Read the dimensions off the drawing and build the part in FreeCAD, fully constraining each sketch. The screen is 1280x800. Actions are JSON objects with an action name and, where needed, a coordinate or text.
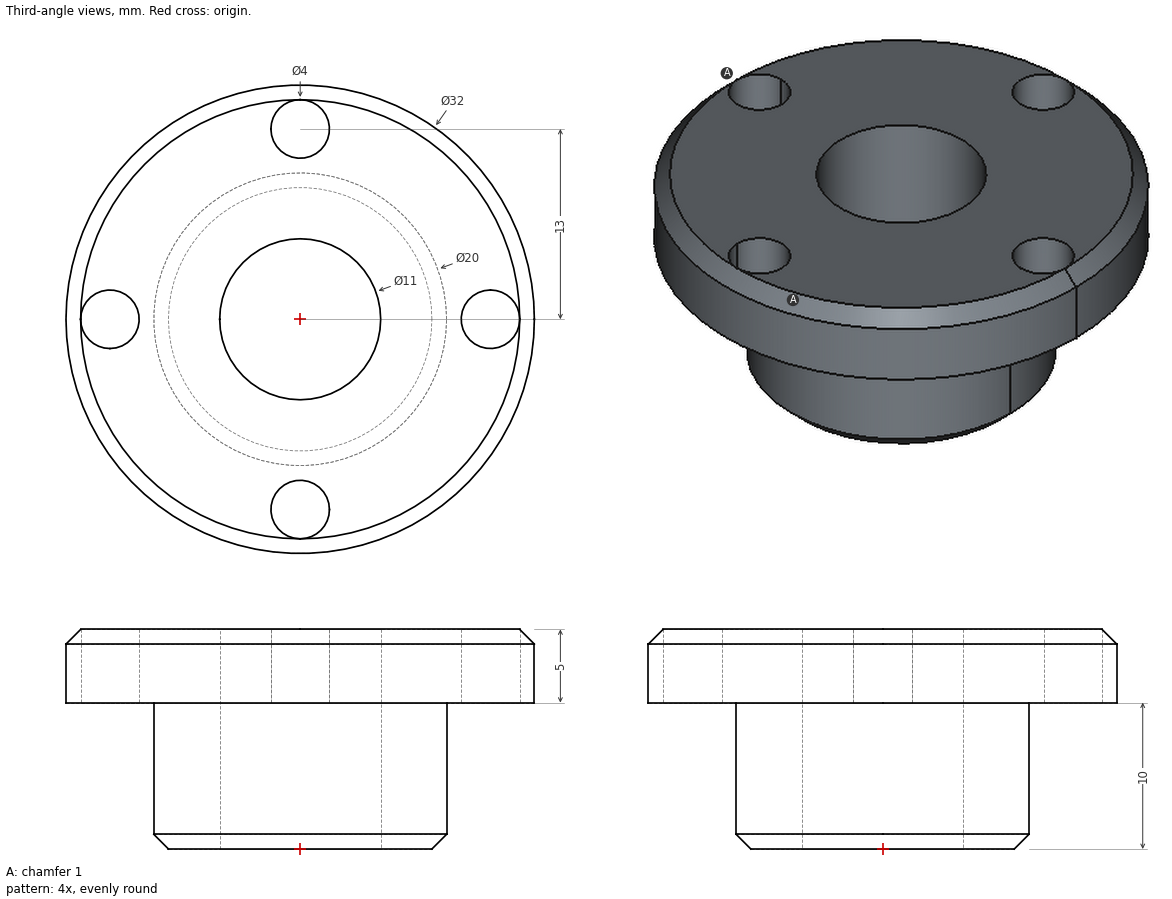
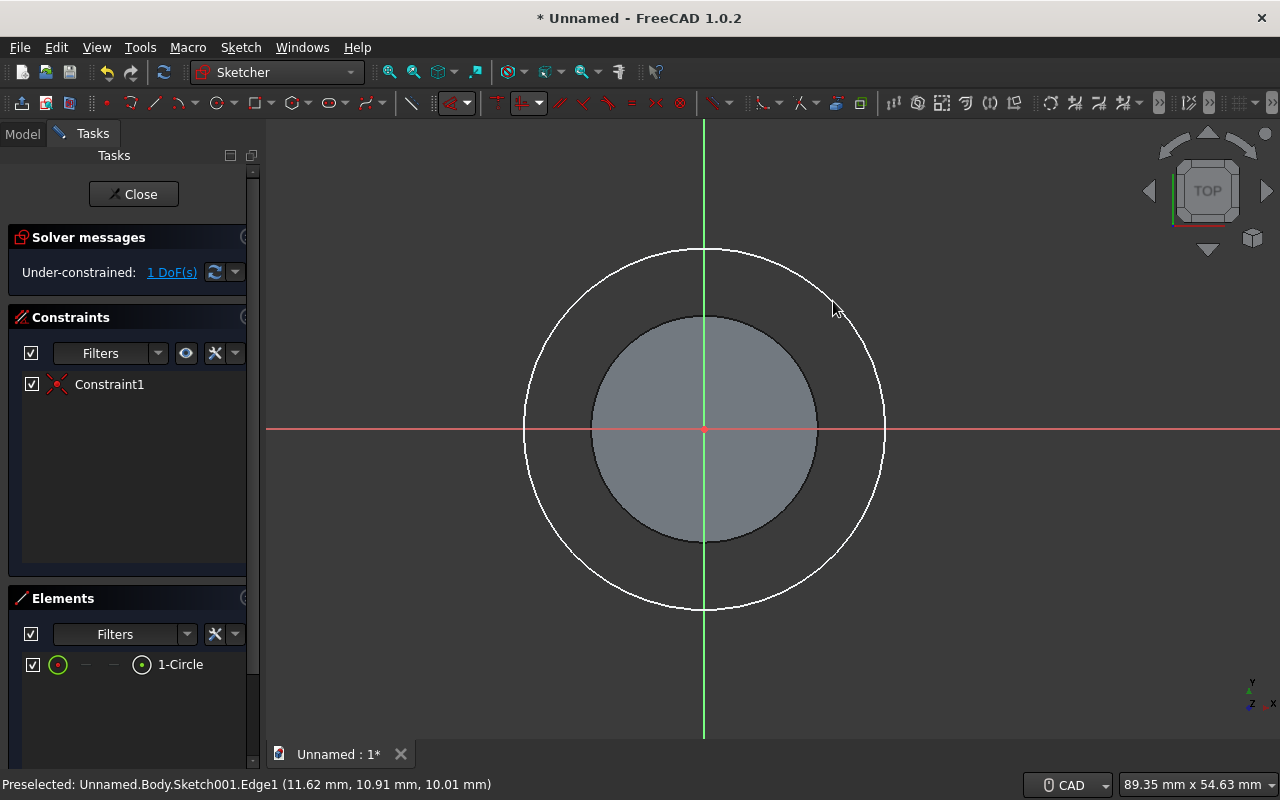
{"action": "left_click", "coordinate": [832, 301]}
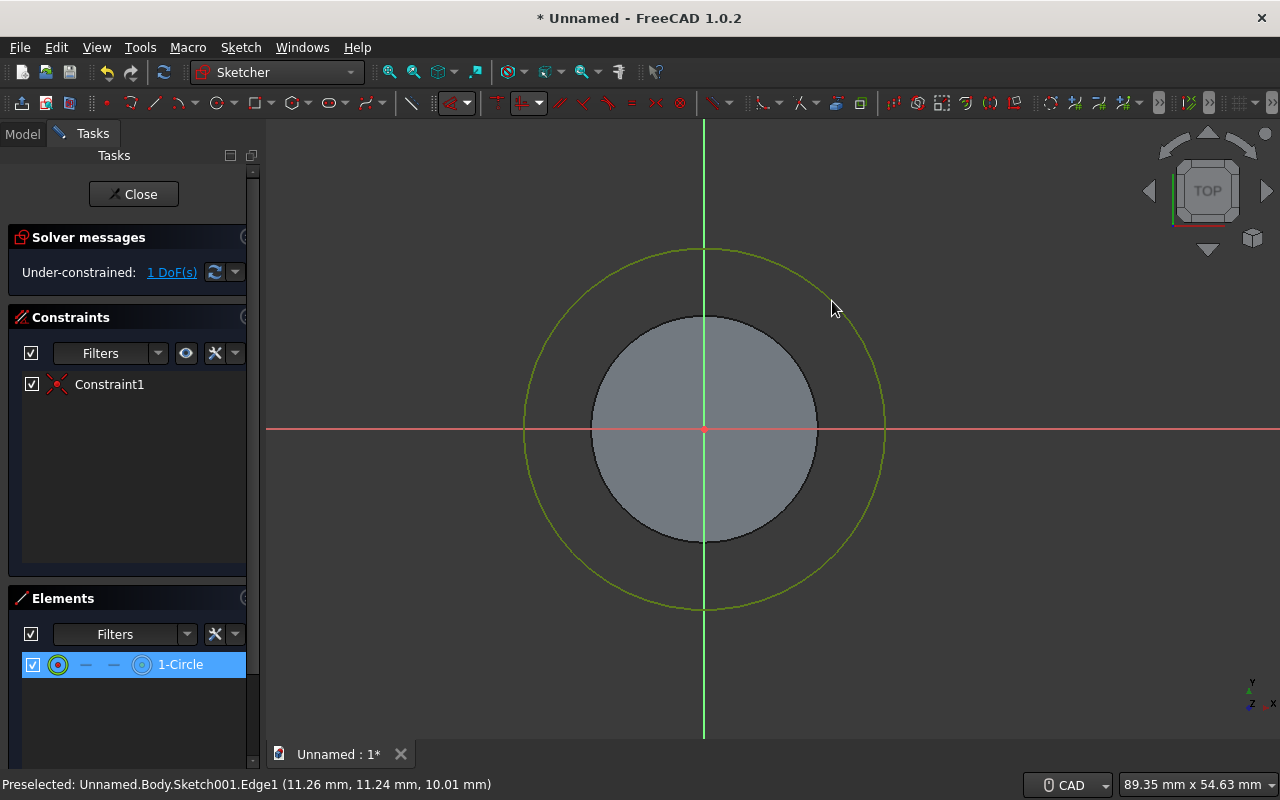
{"action": "key", "text": "k o"}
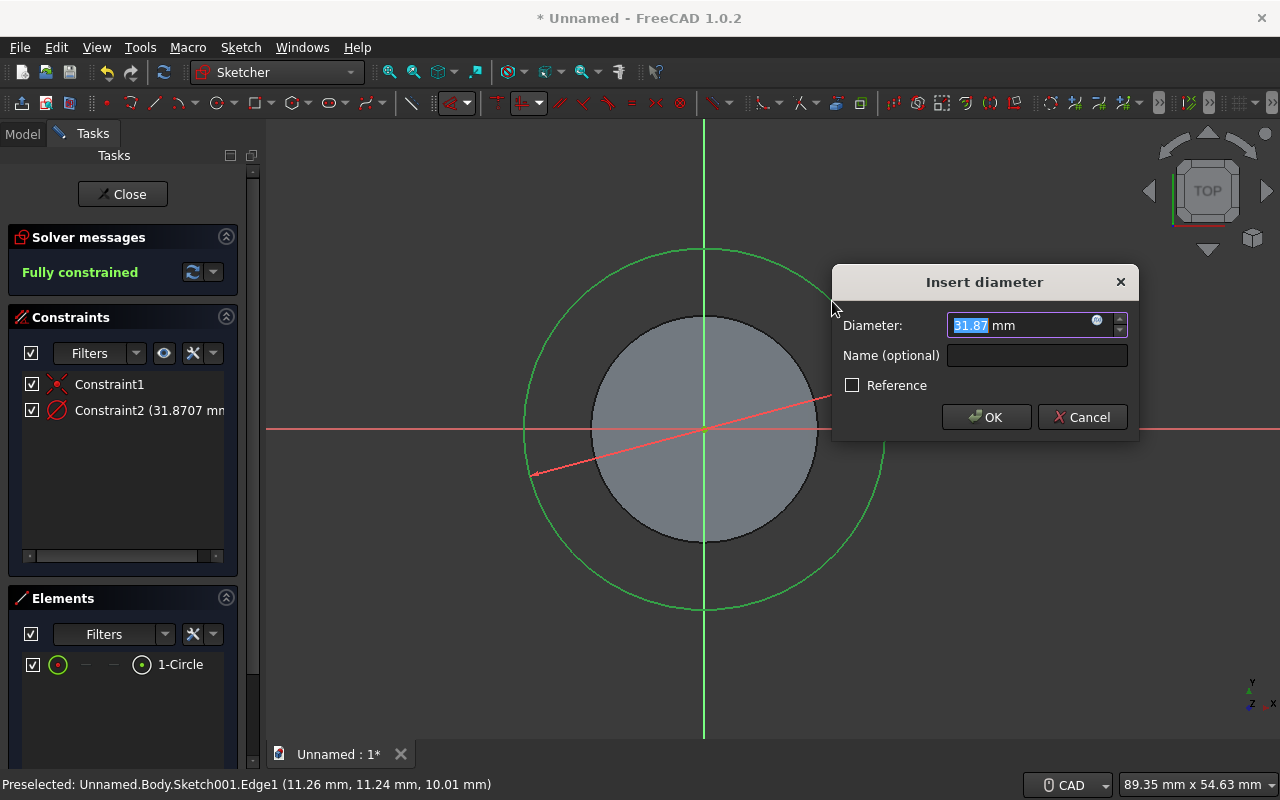
{"action": "type", "text": "32"}
{"action": "key", "text": "Return"}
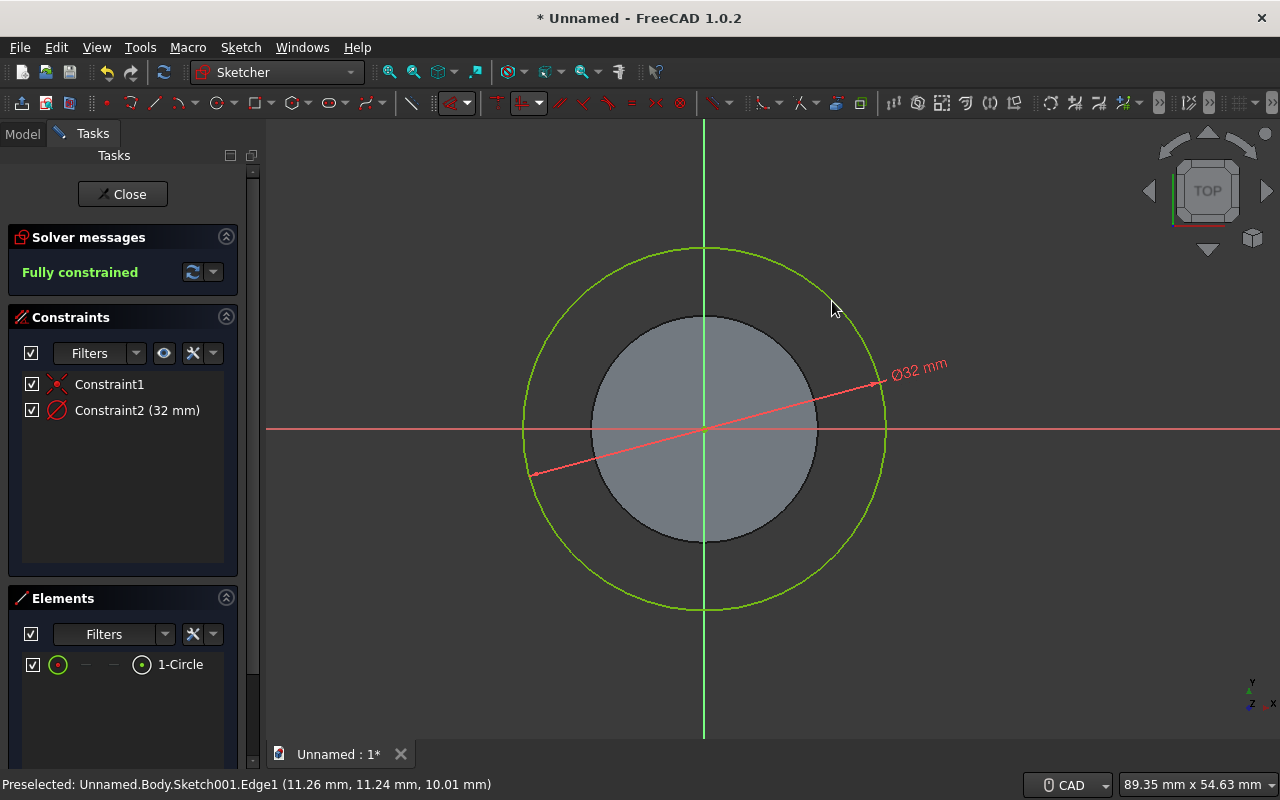
{"action": "left_click", "coordinate": [123, 194]}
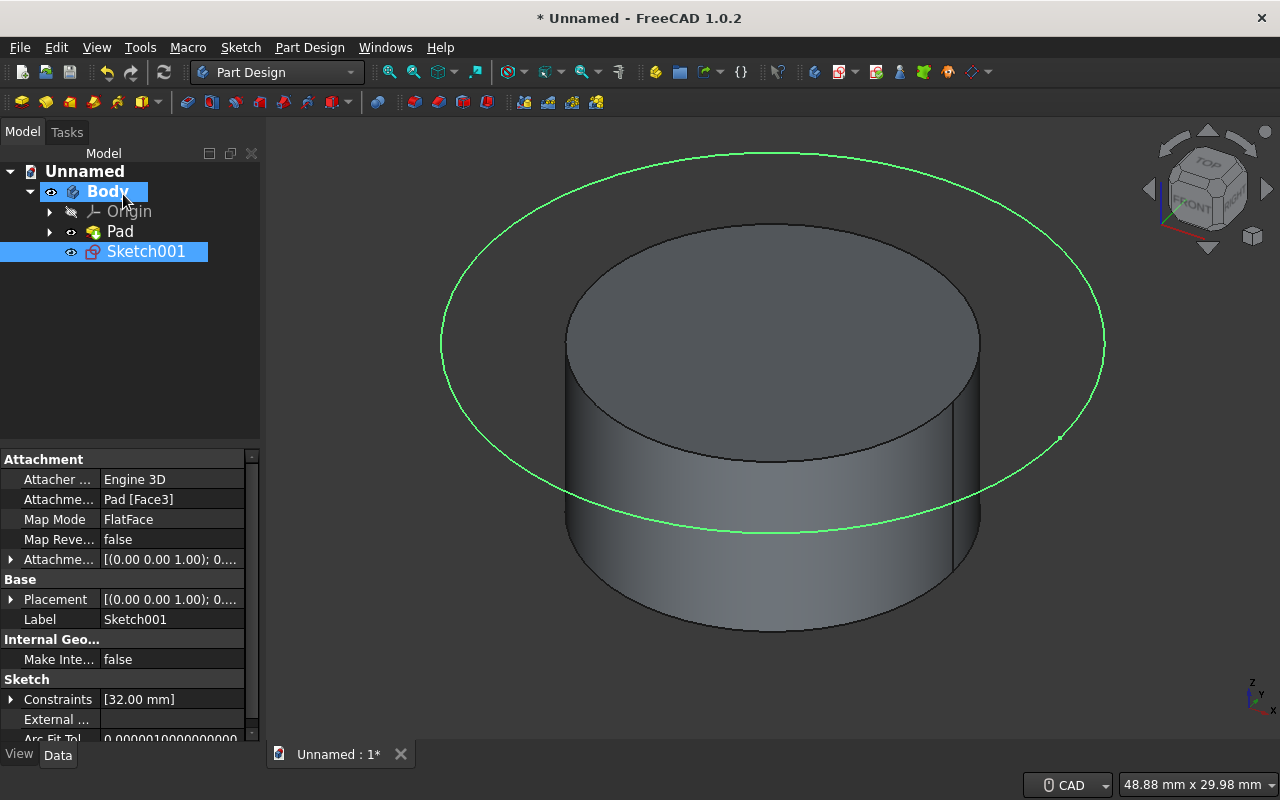
{"action": "left_click", "coordinate": [22, 102]}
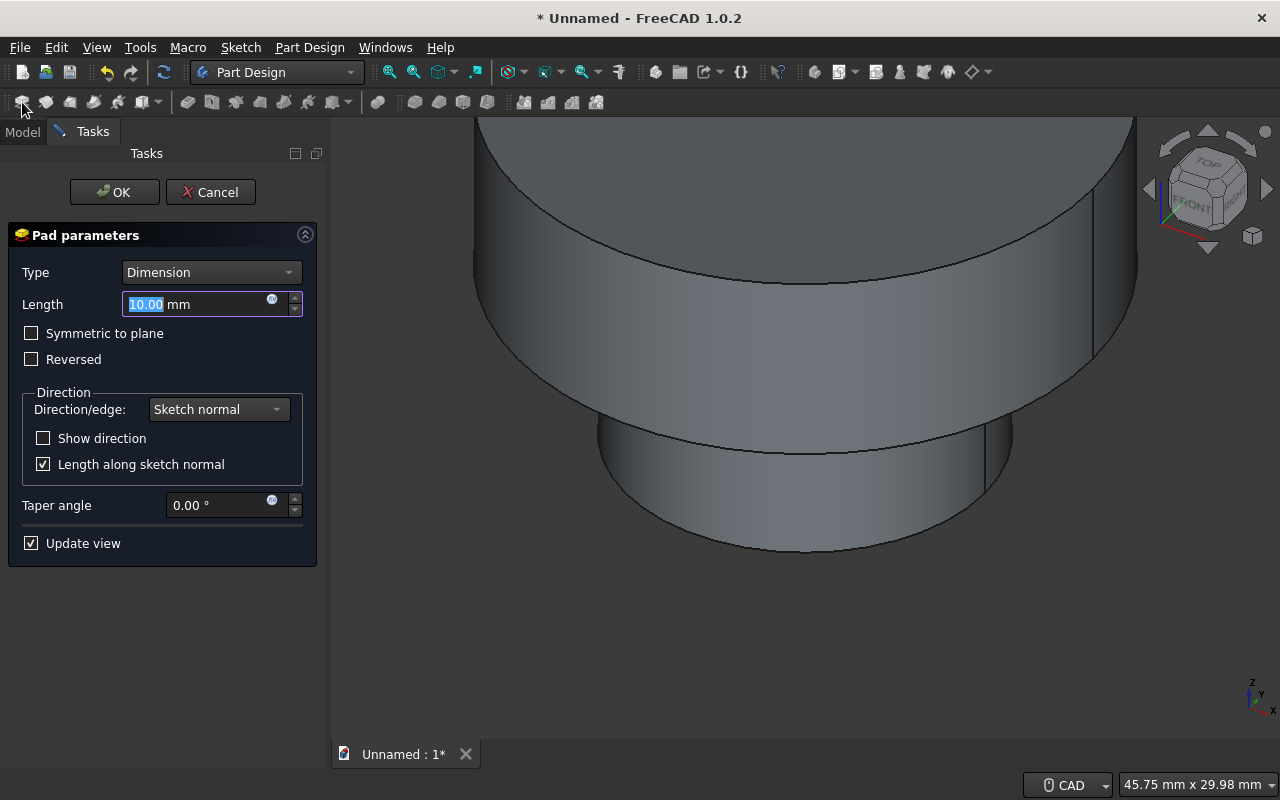
{"action": "type", "text": "5"}
{"action": "key", "text": "Tab"}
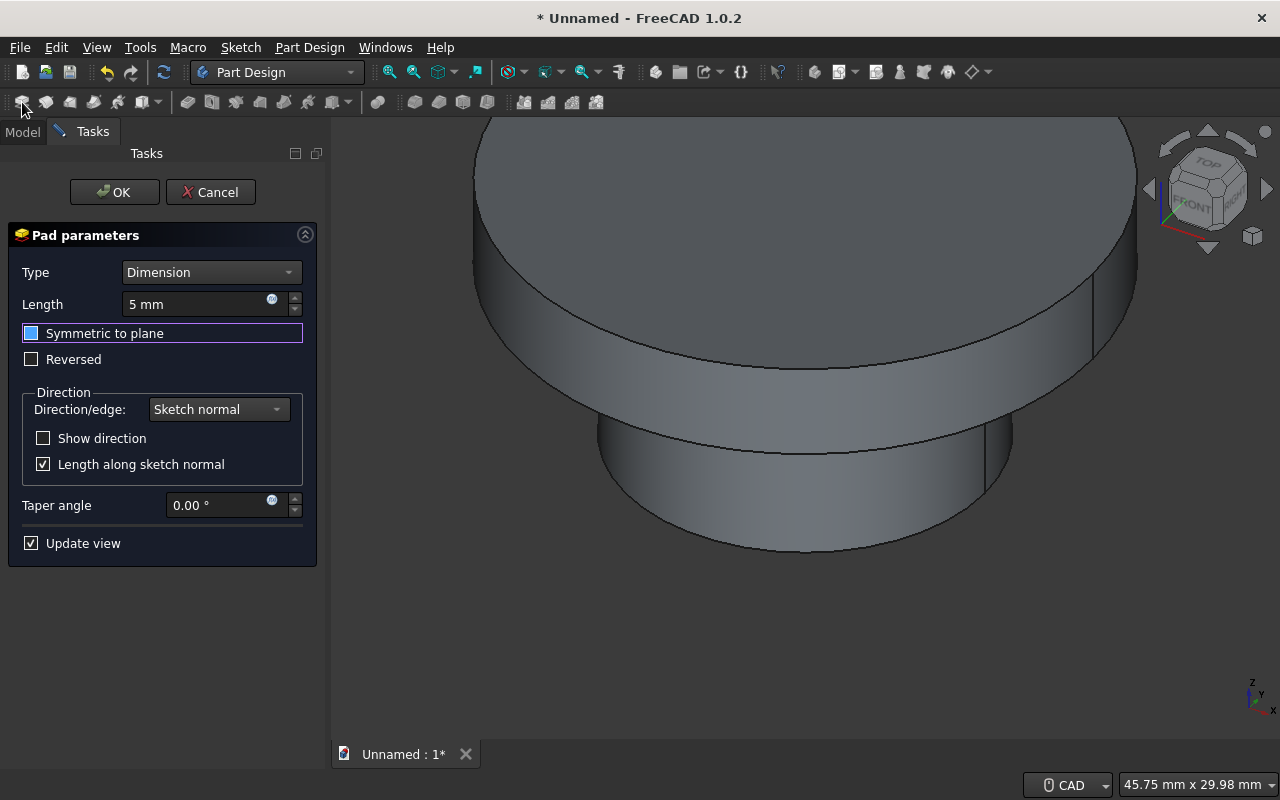
{"action": "left_click", "coordinate": [115, 192]}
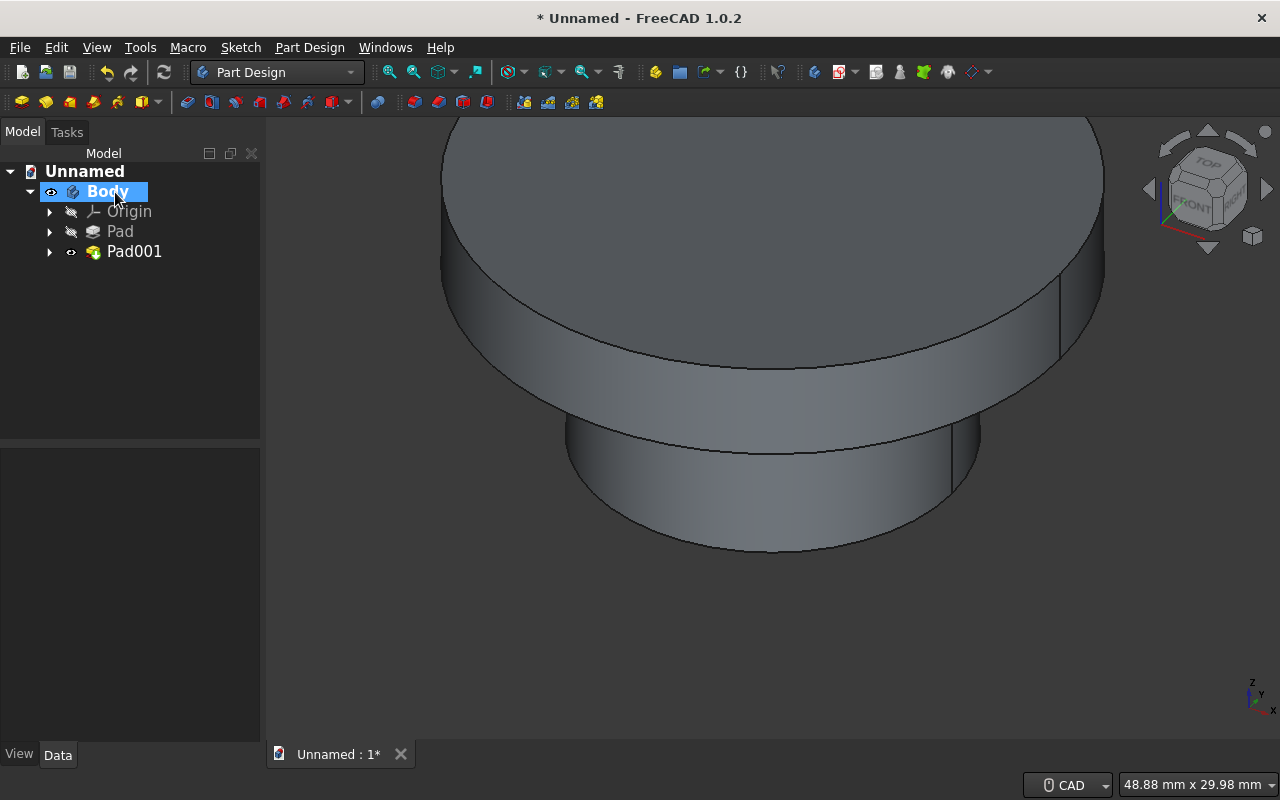
{"action": "key", "text": "v f"}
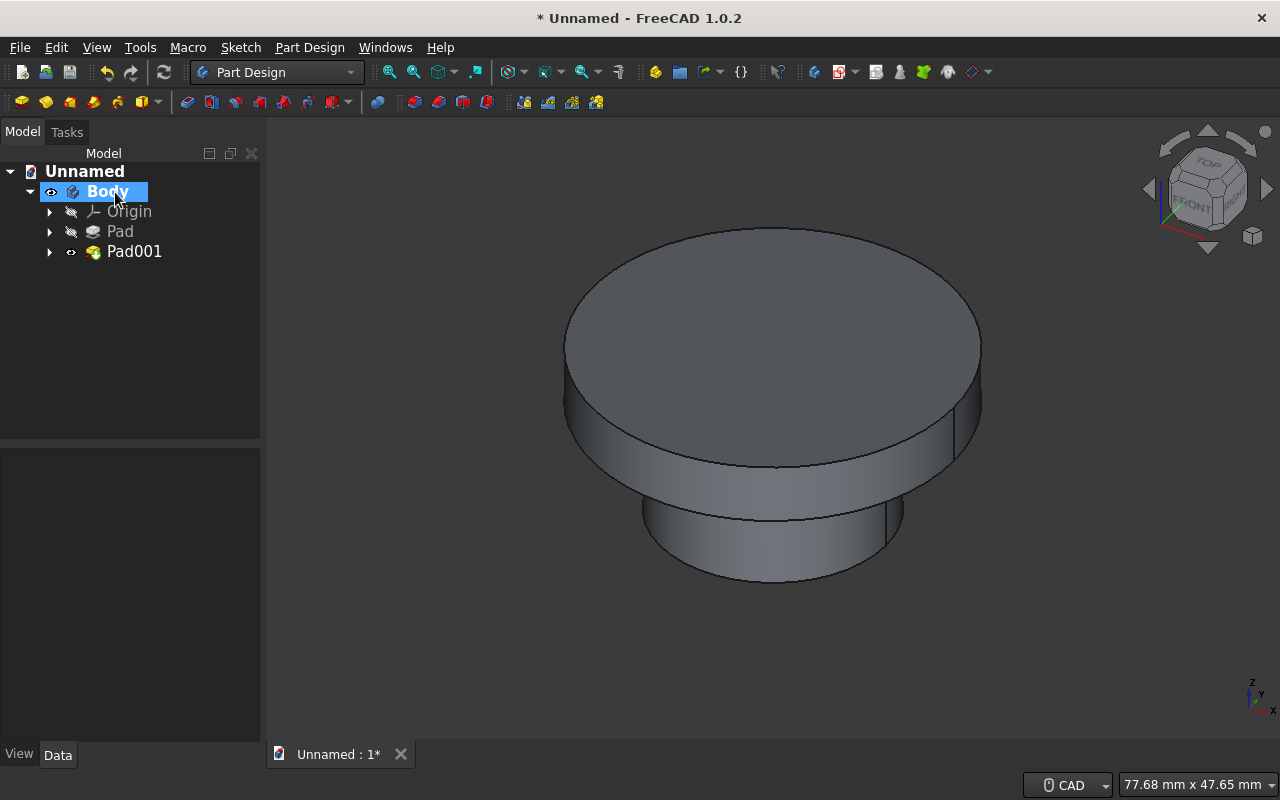
{"action": "left_click", "coordinate": [896, 532]}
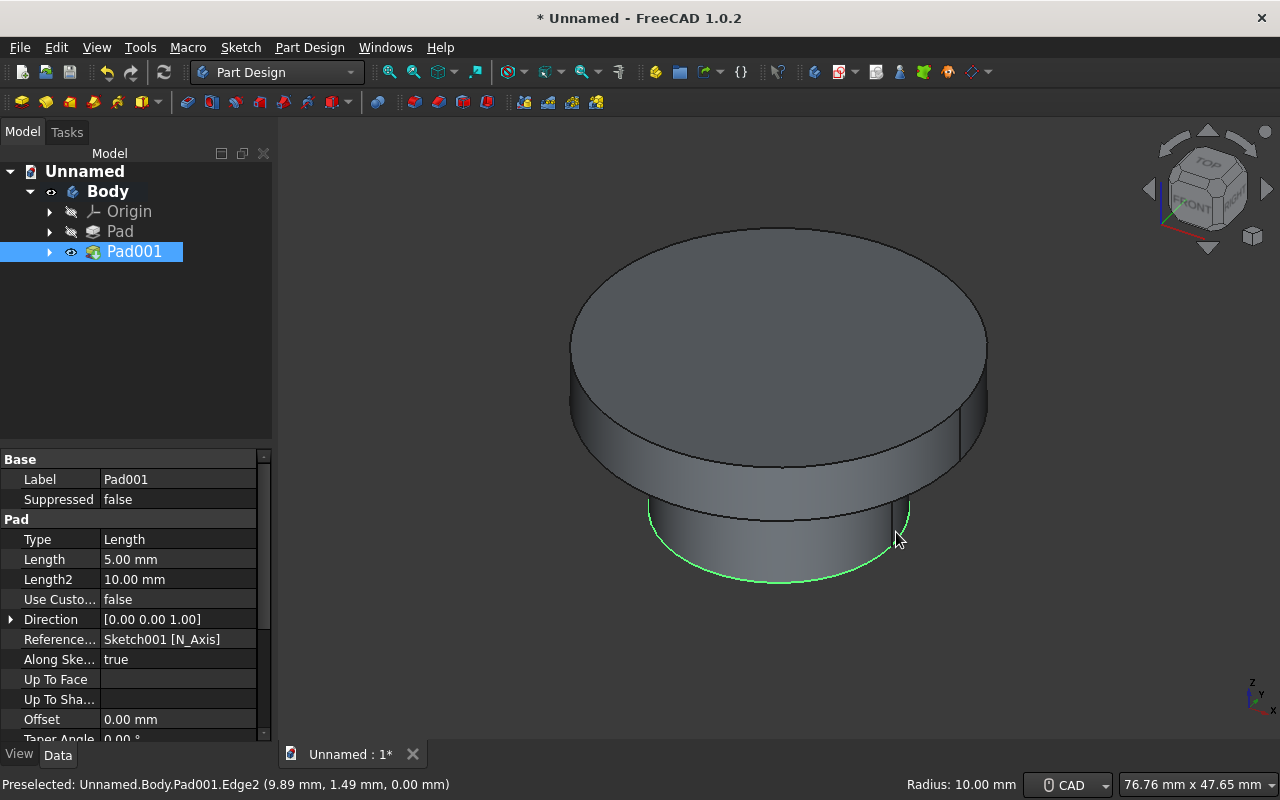
{"action": "left_click", "coordinate": [571, 359], "text": "ctrl"}